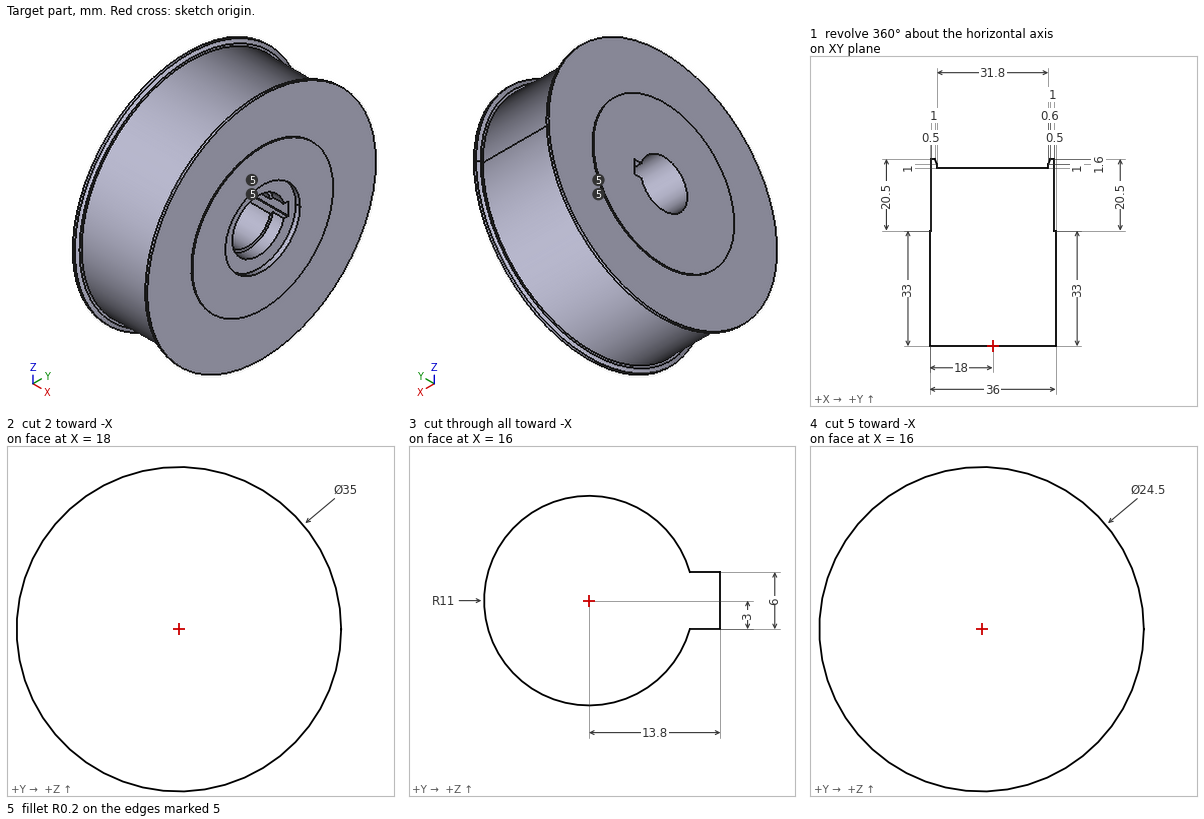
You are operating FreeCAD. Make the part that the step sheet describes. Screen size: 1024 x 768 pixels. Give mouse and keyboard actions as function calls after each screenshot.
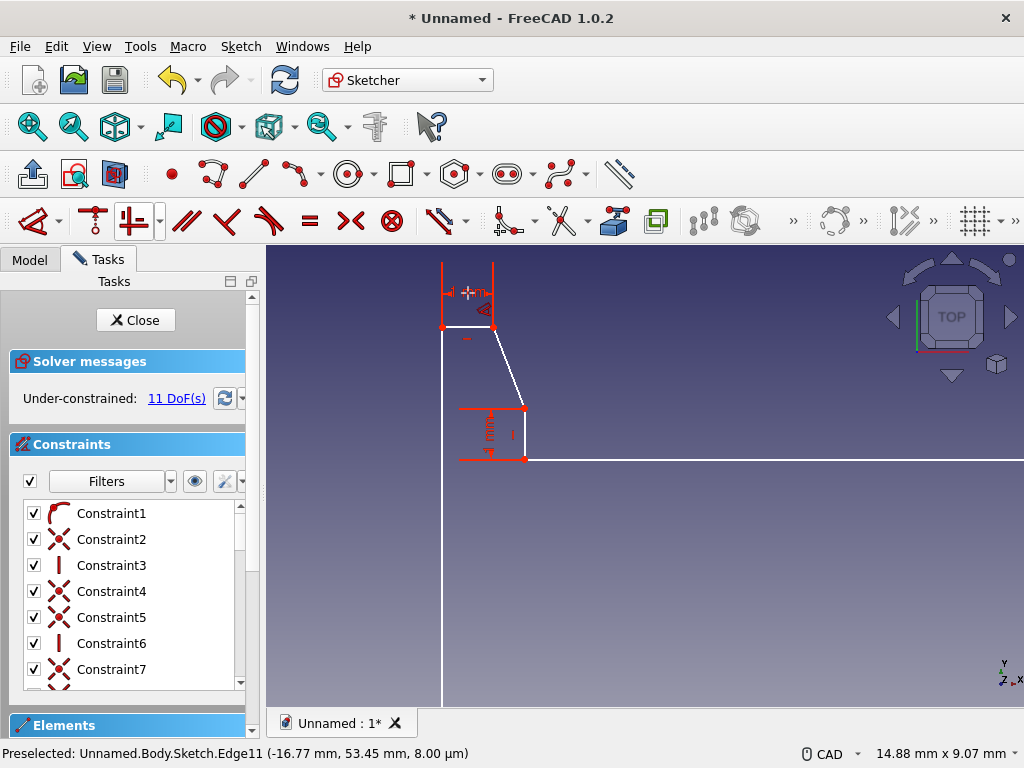
scroll(482, 325, down, 11)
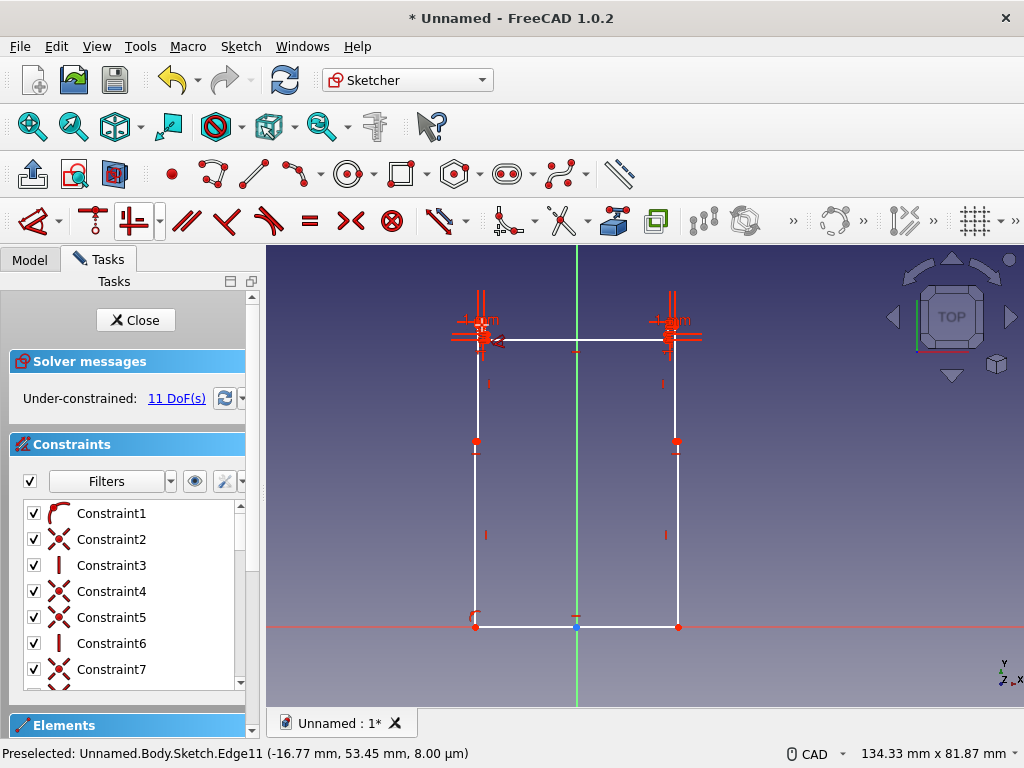
click(536, 627)
click(530, 661)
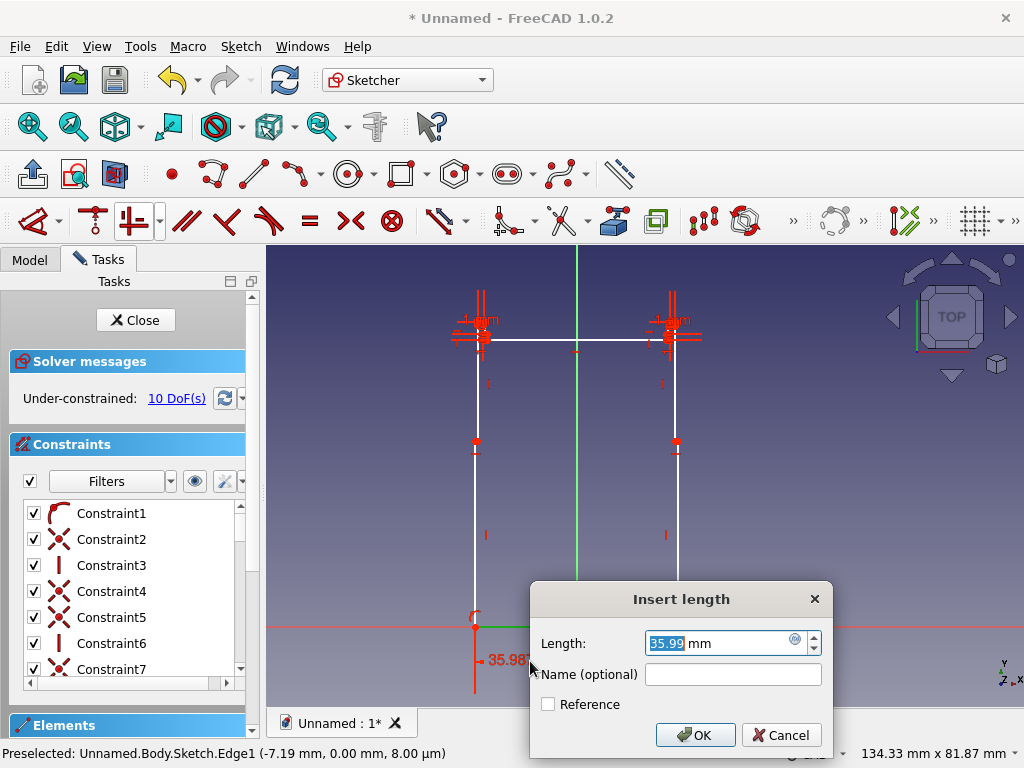
text(36)
key(Return)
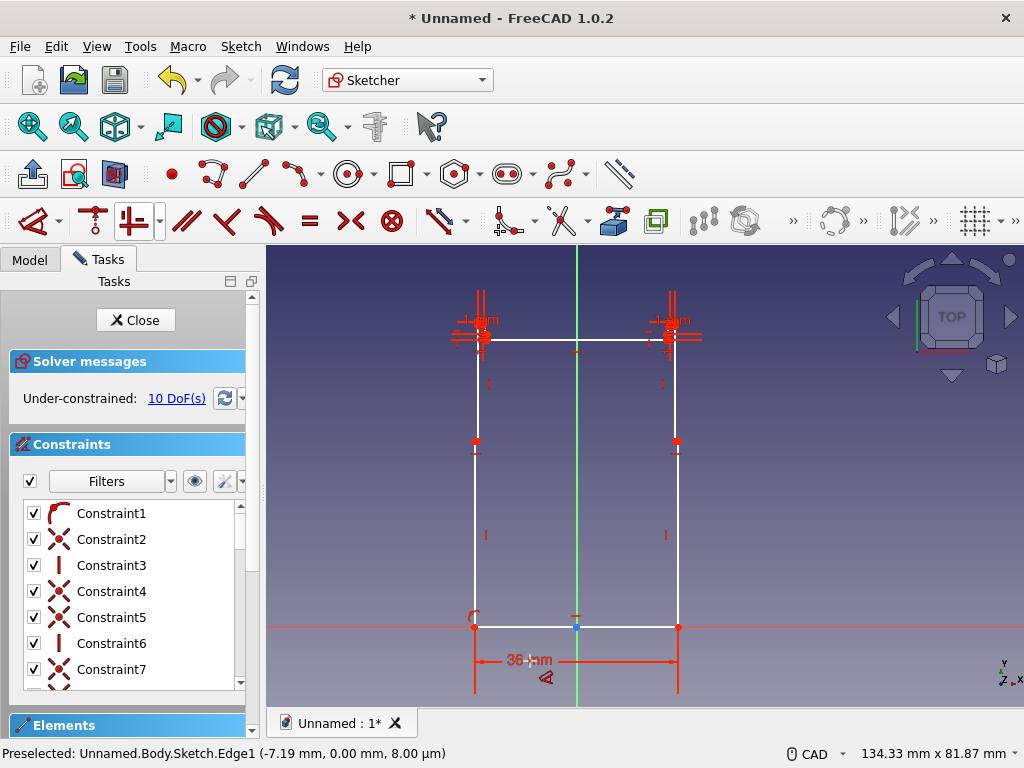
click(678, 572)
click(712, 535)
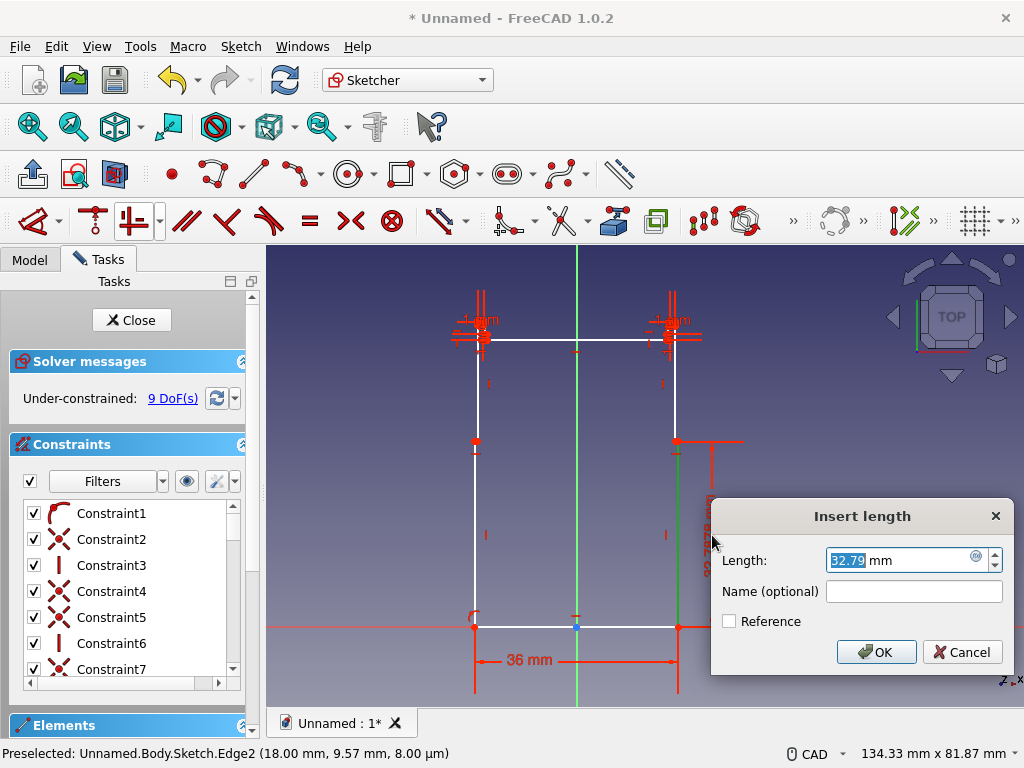
text(33)
key(Return)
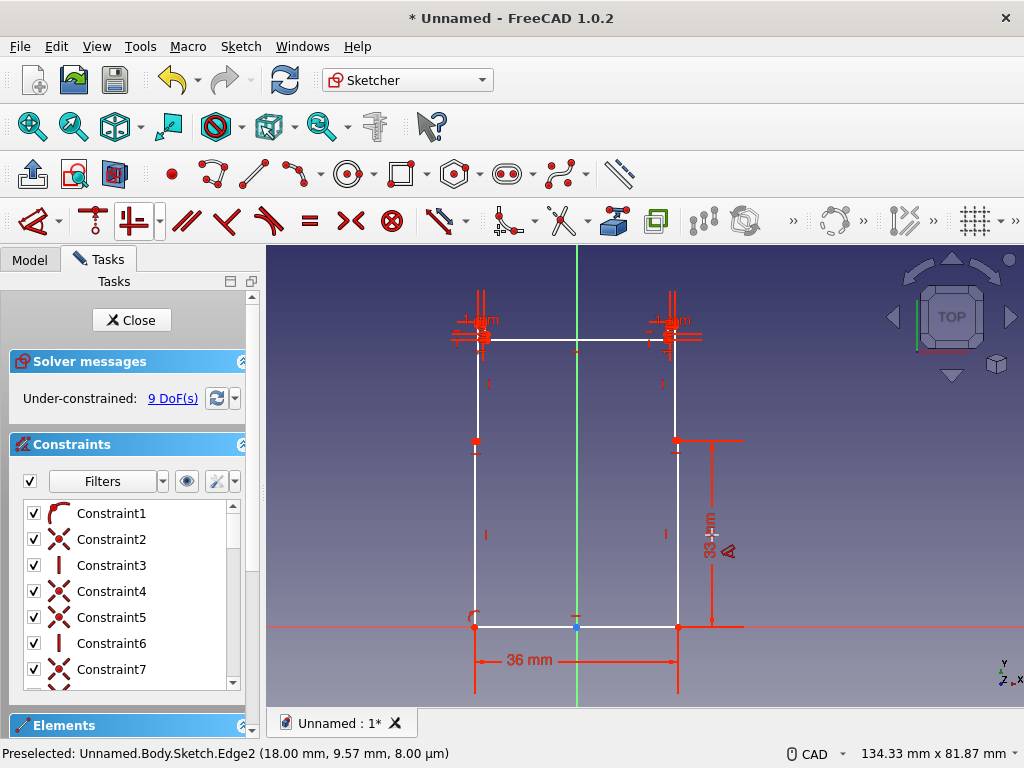
click(475, 498)
click(441, 535)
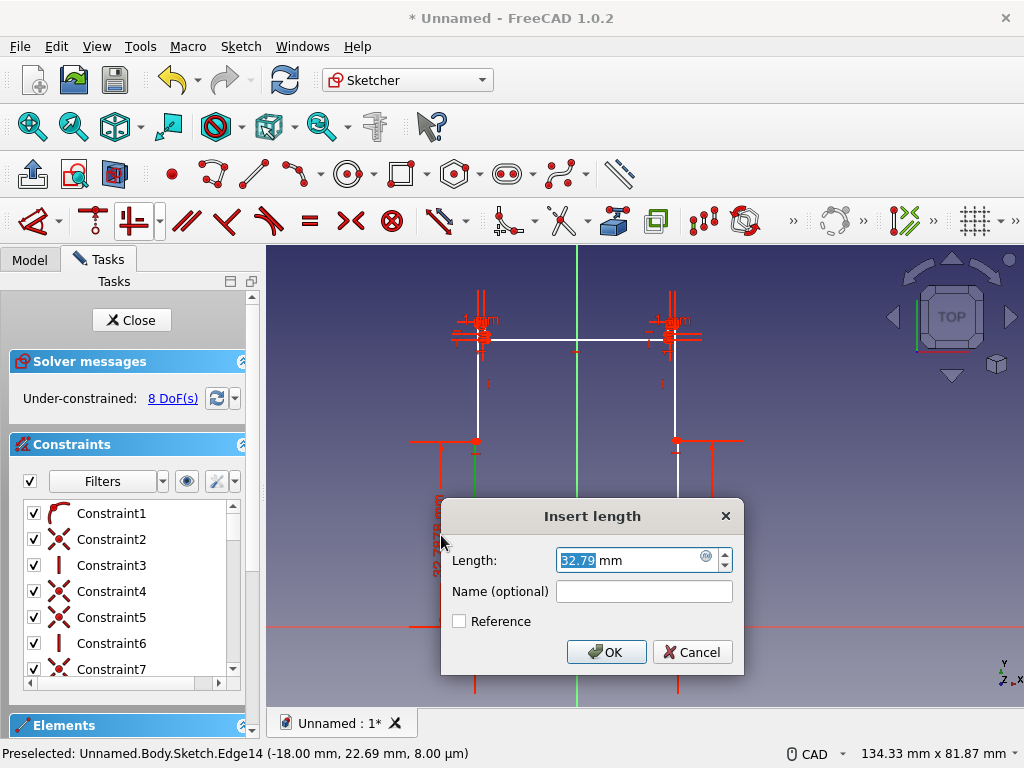
text(33)
key(Return)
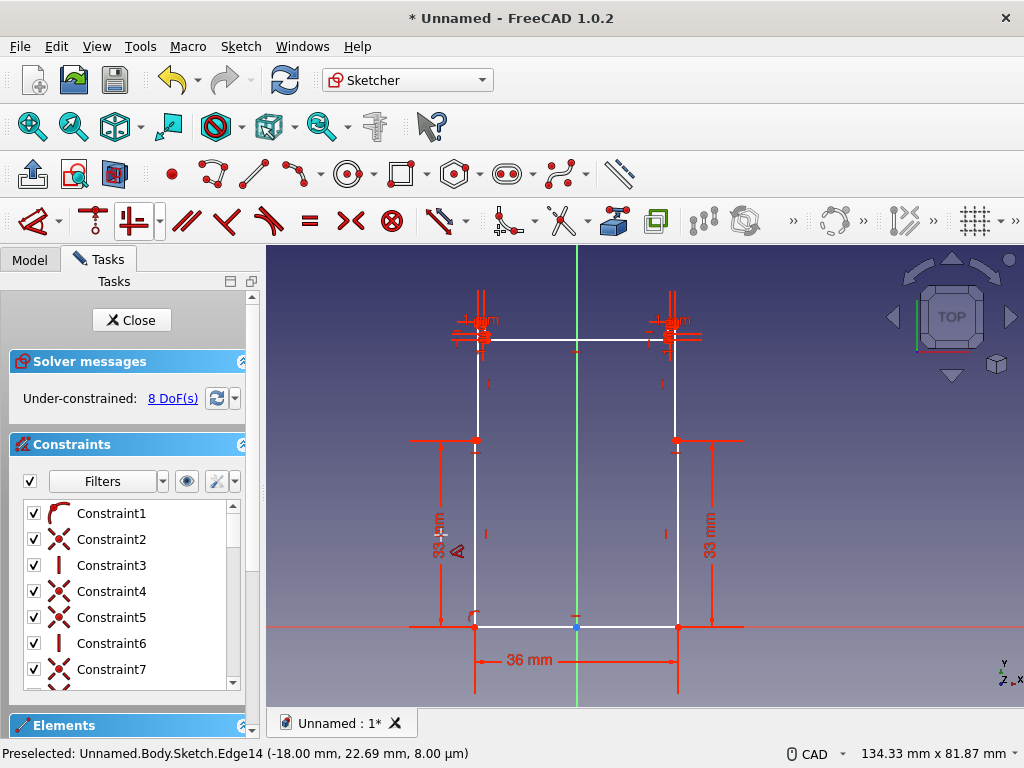
scroll(677, 441, up, 14)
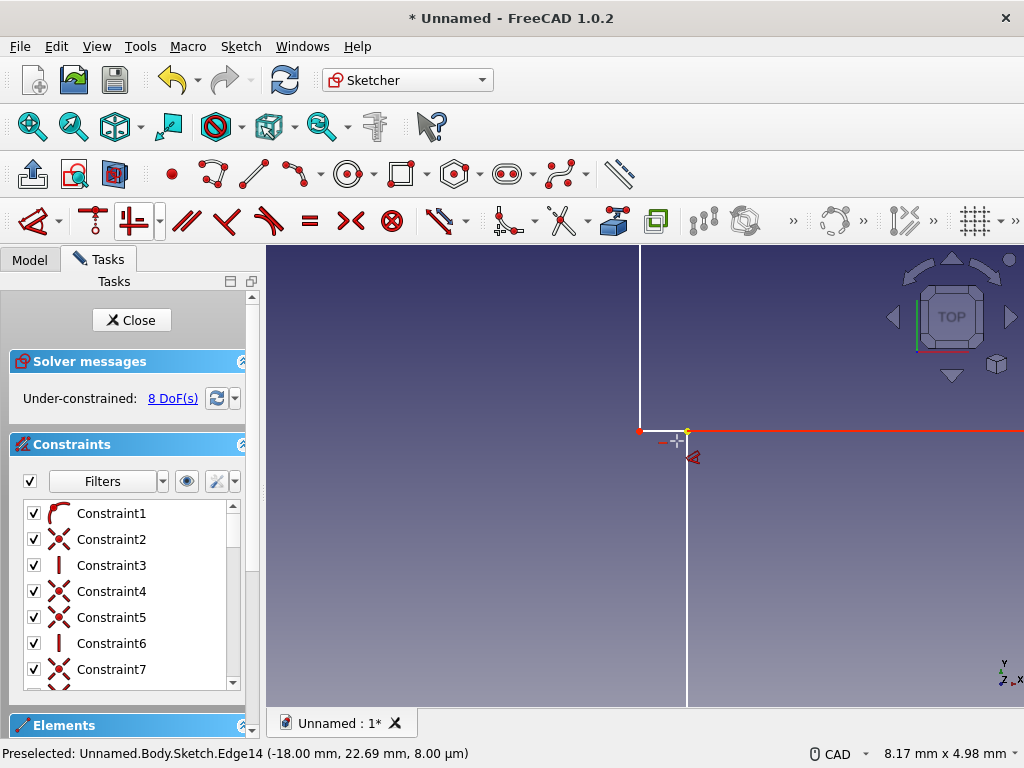
click(664, 431)
click(664, 397)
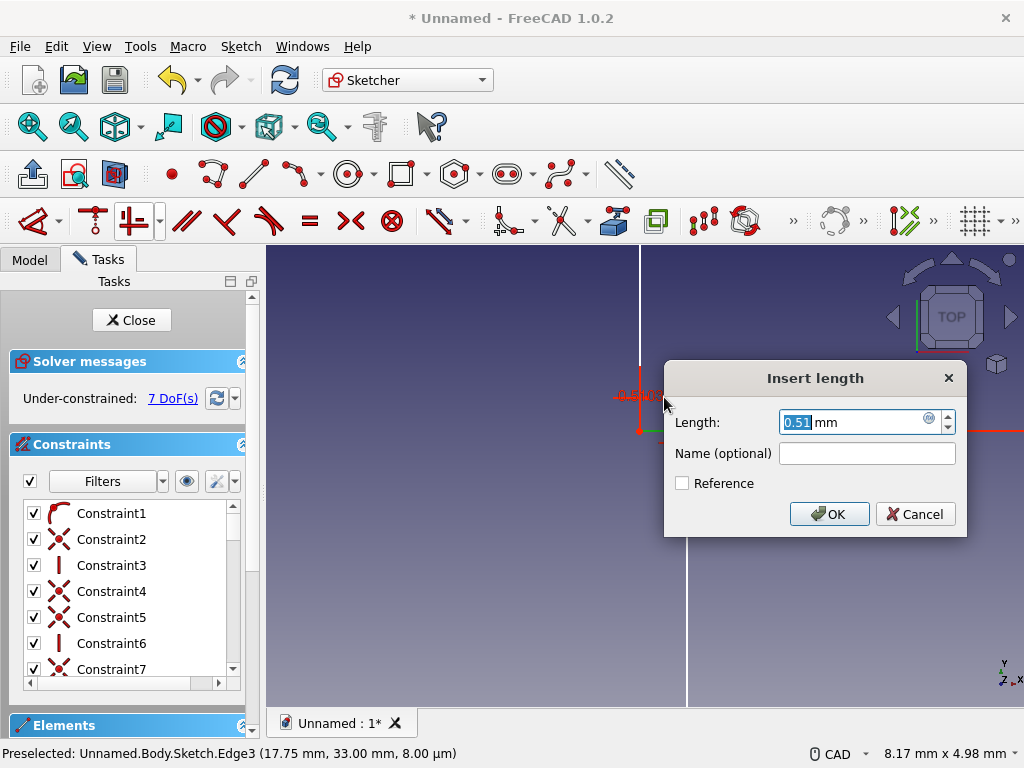
text(0.5)
key(Return)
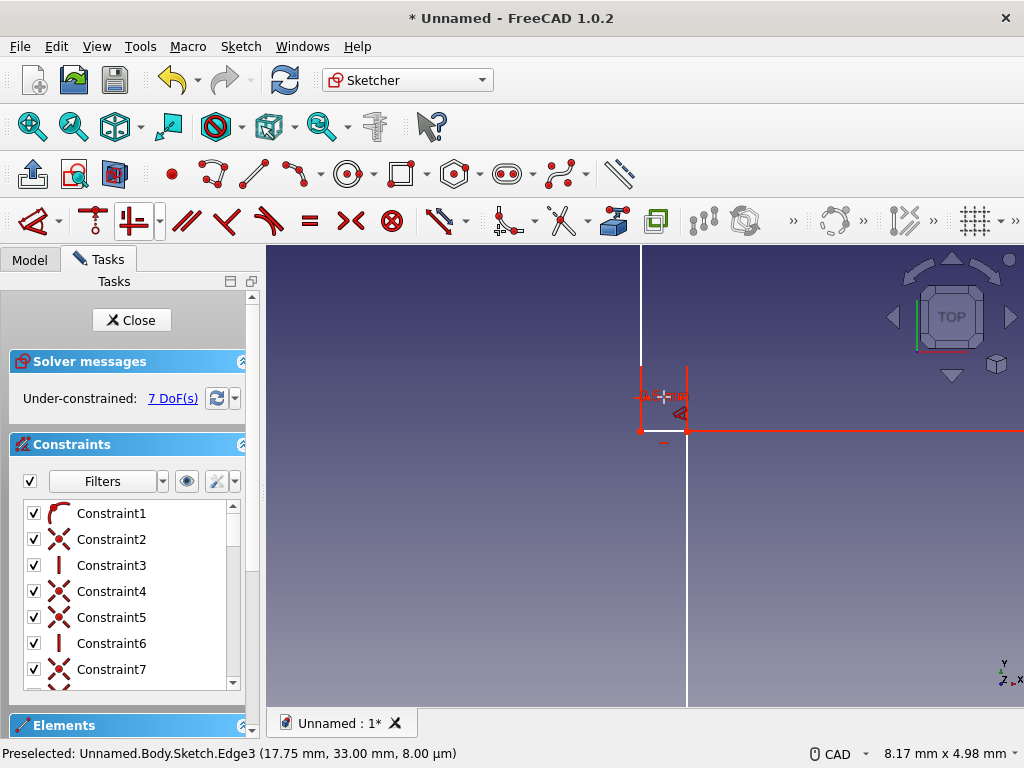
scroll(677, 441, down, 14)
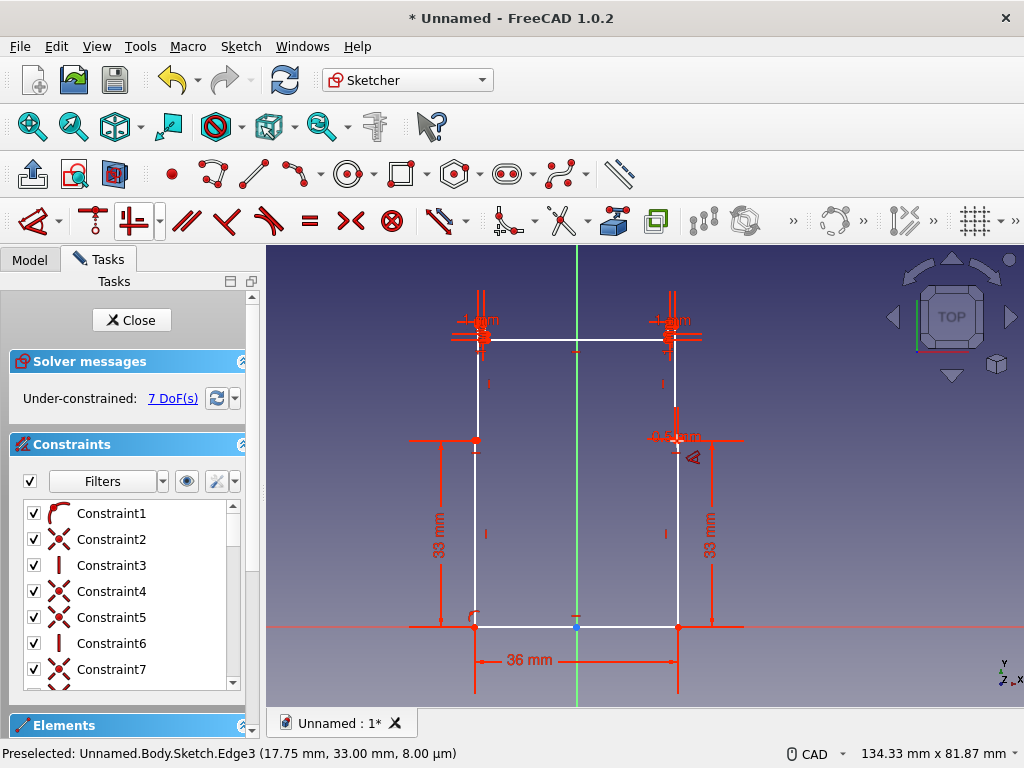
scroll(477, 441, up, 14)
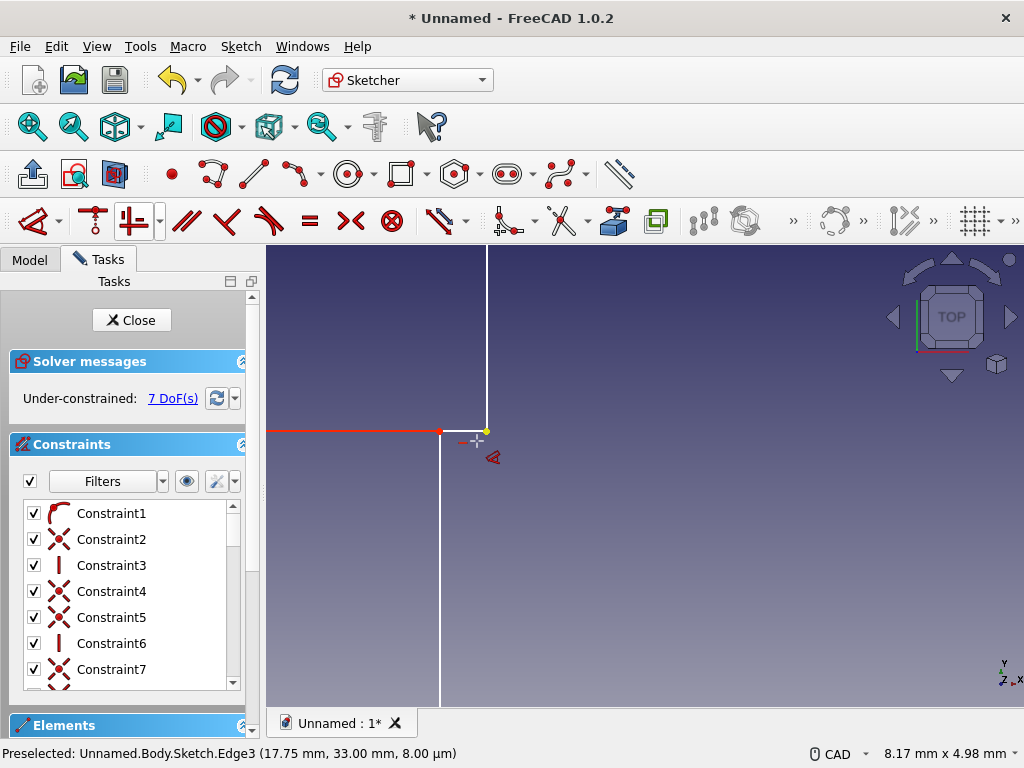
click(473, 431)
click(463, 397)